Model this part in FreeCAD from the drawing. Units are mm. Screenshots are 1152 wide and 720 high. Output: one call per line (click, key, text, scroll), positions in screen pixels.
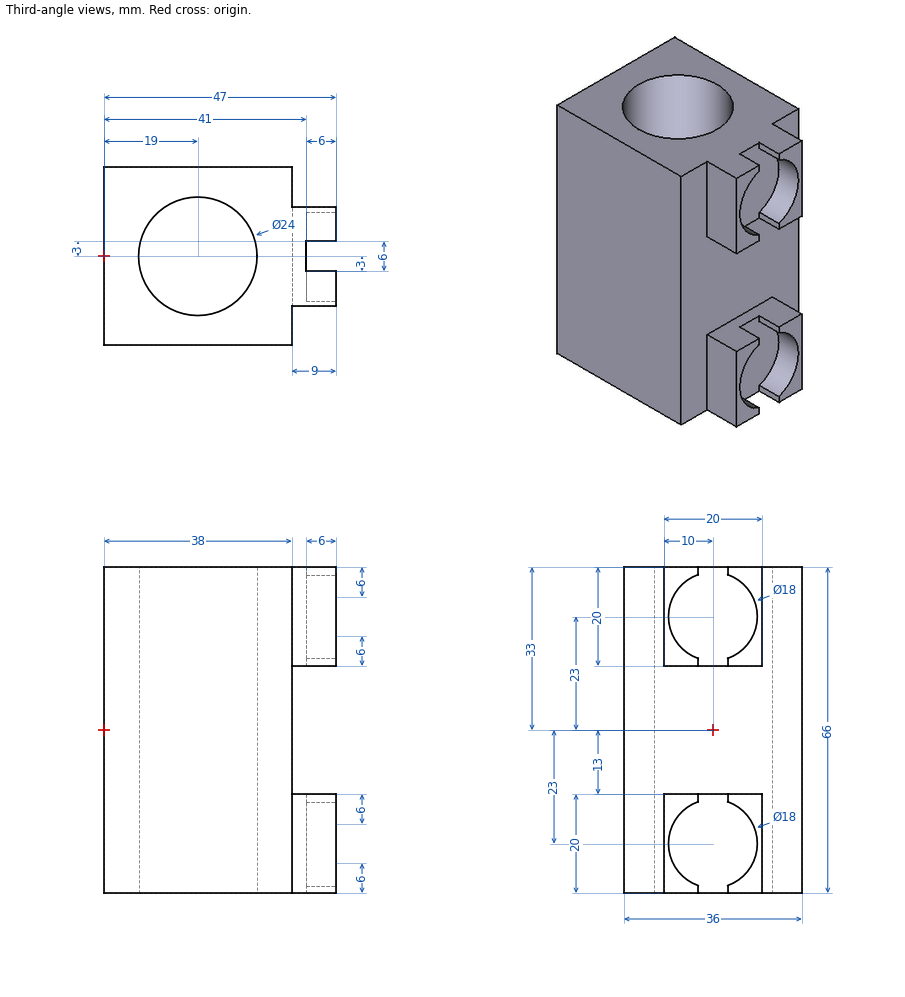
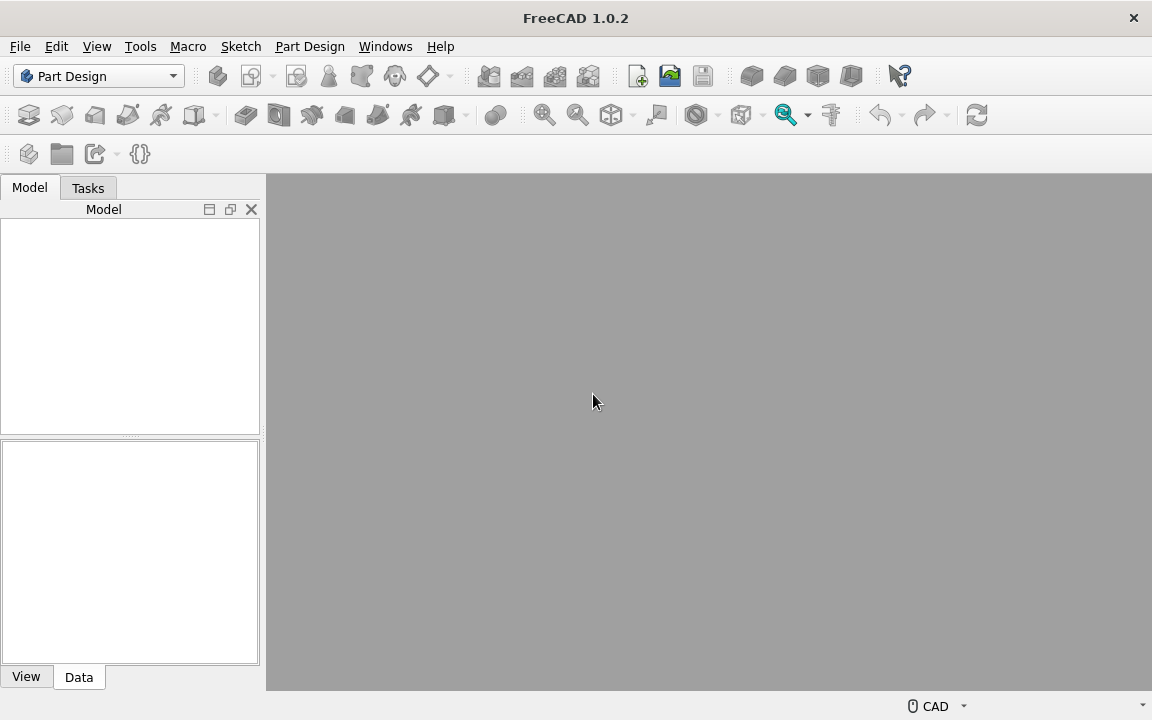
key(ctrl+n)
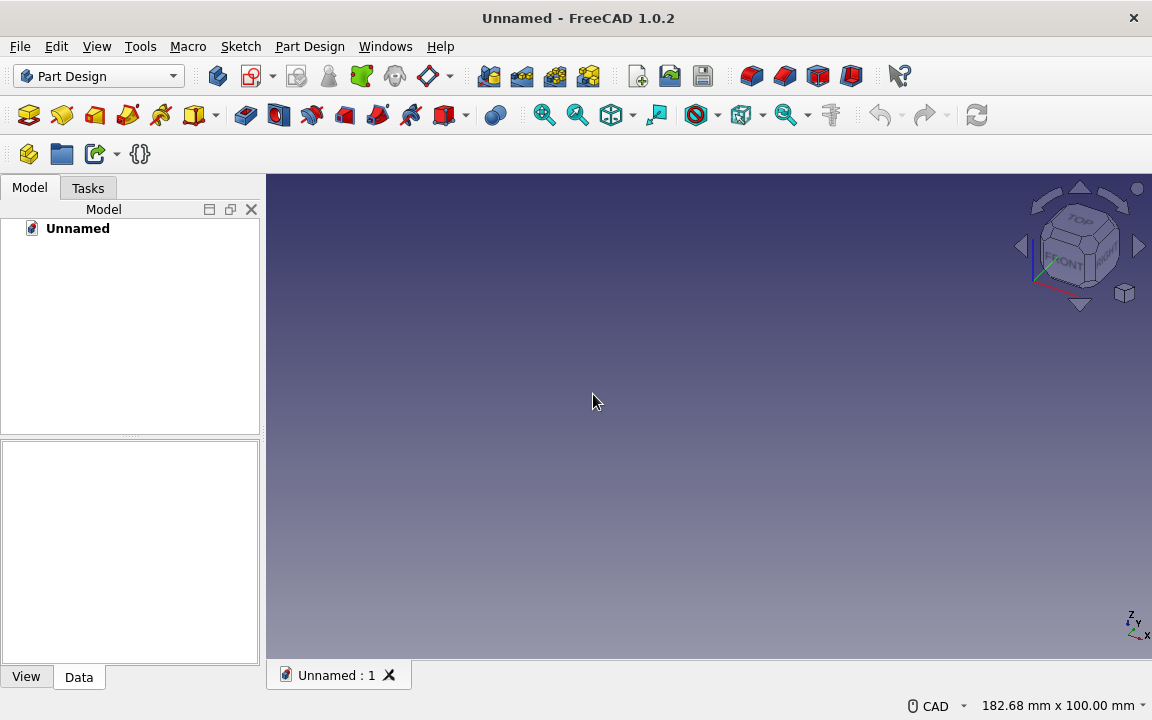
click(250, 76)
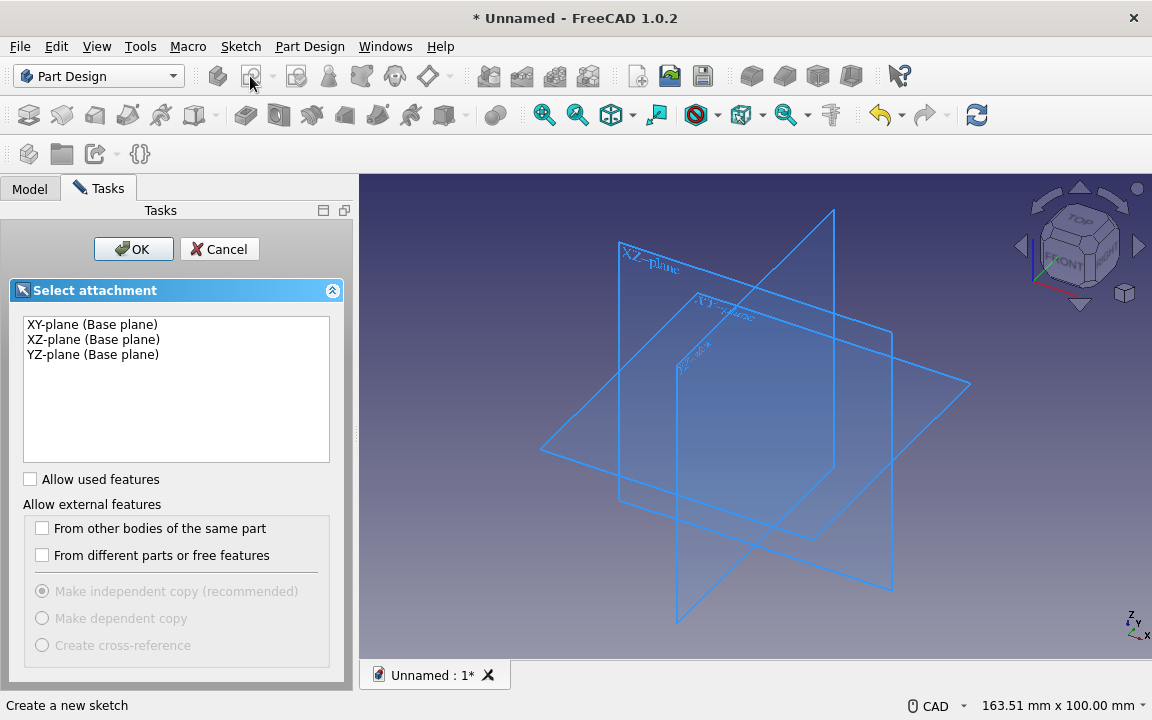
click(84, 354)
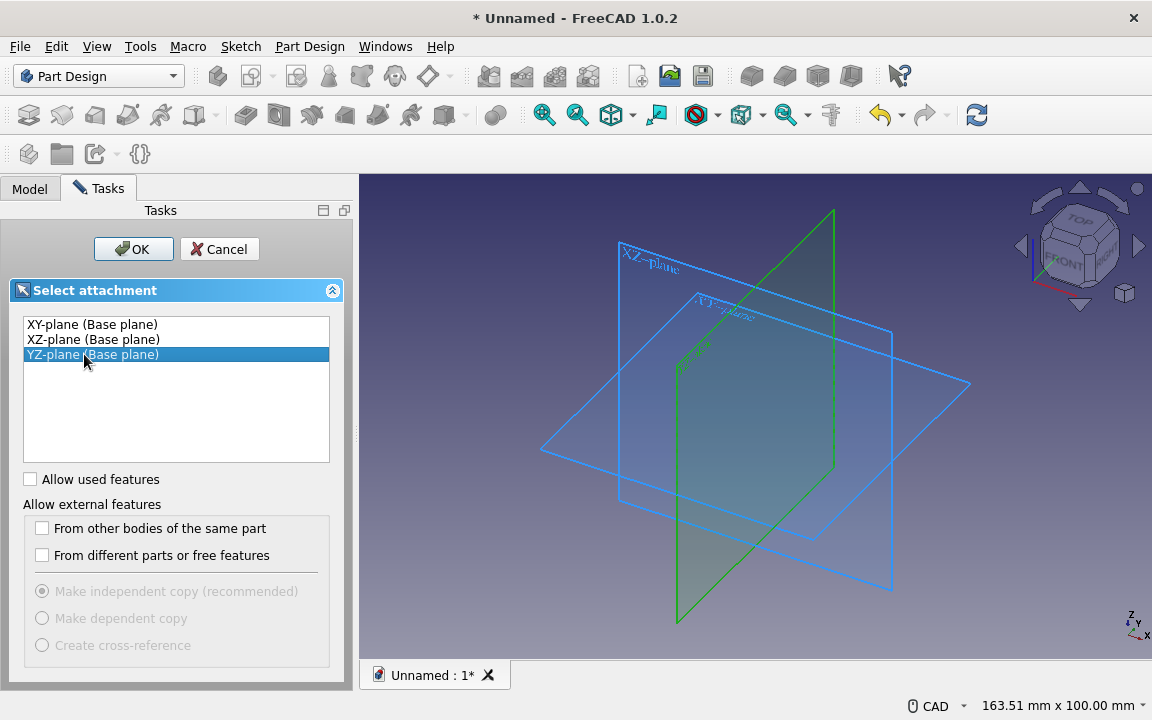
click(134, 249)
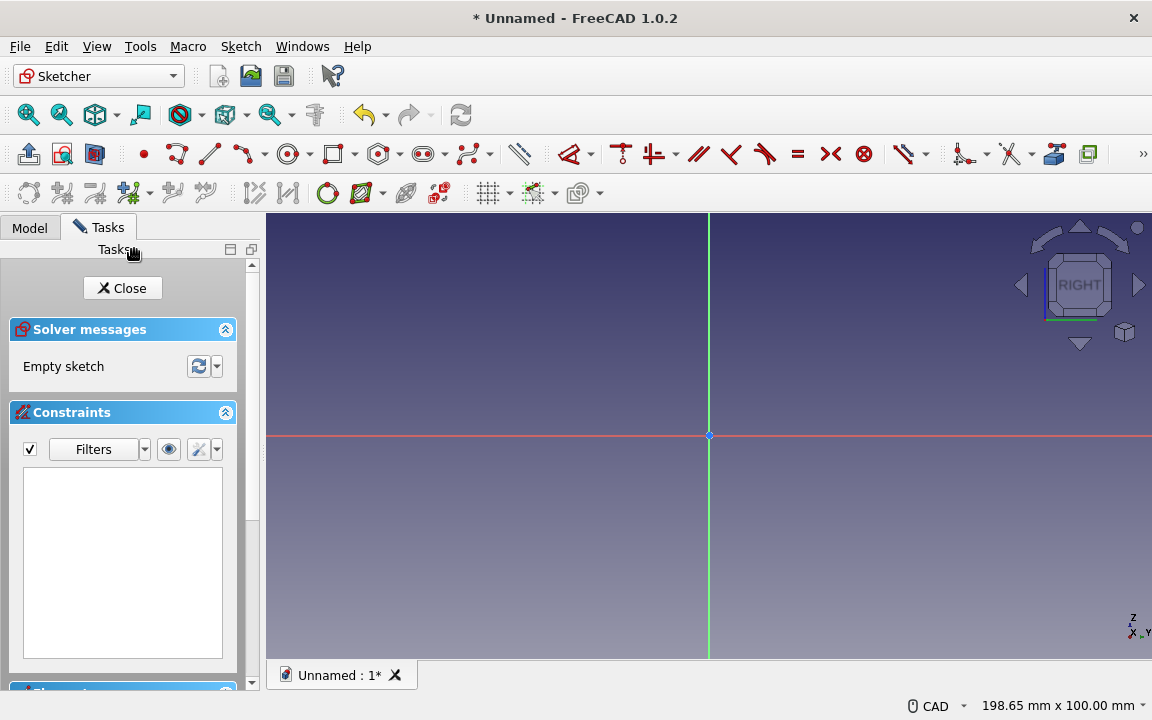
key(g)
key(v)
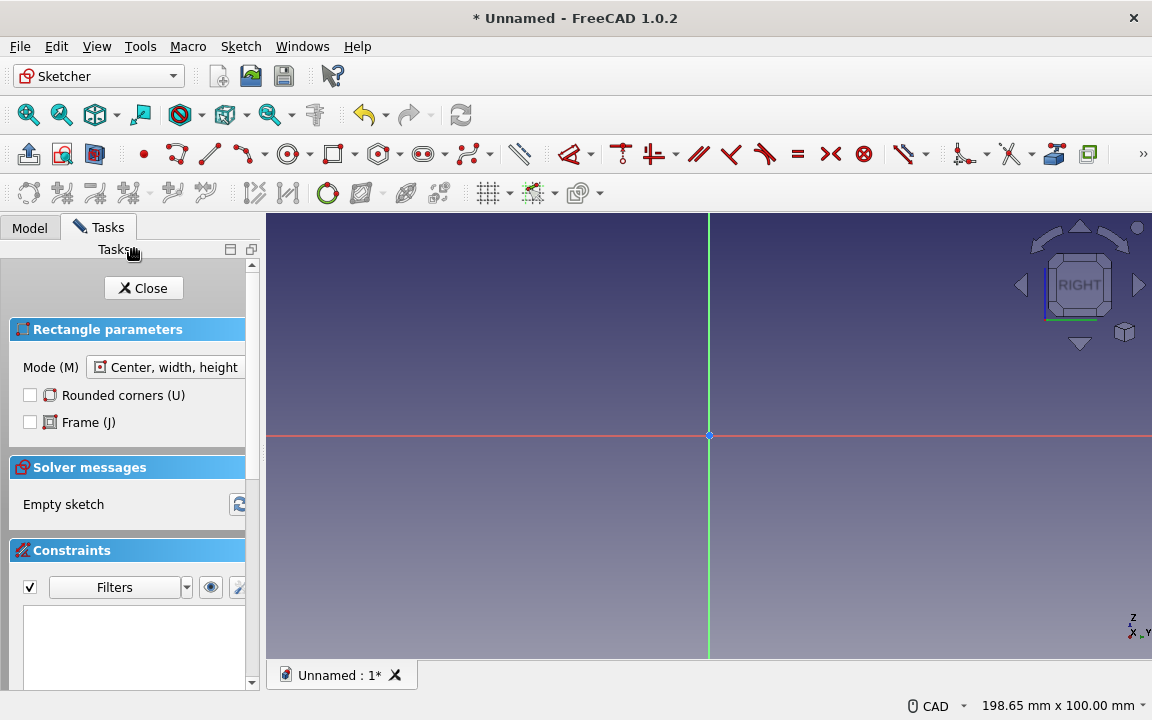
click(709, 436)
click(789, 289)
key(Escape)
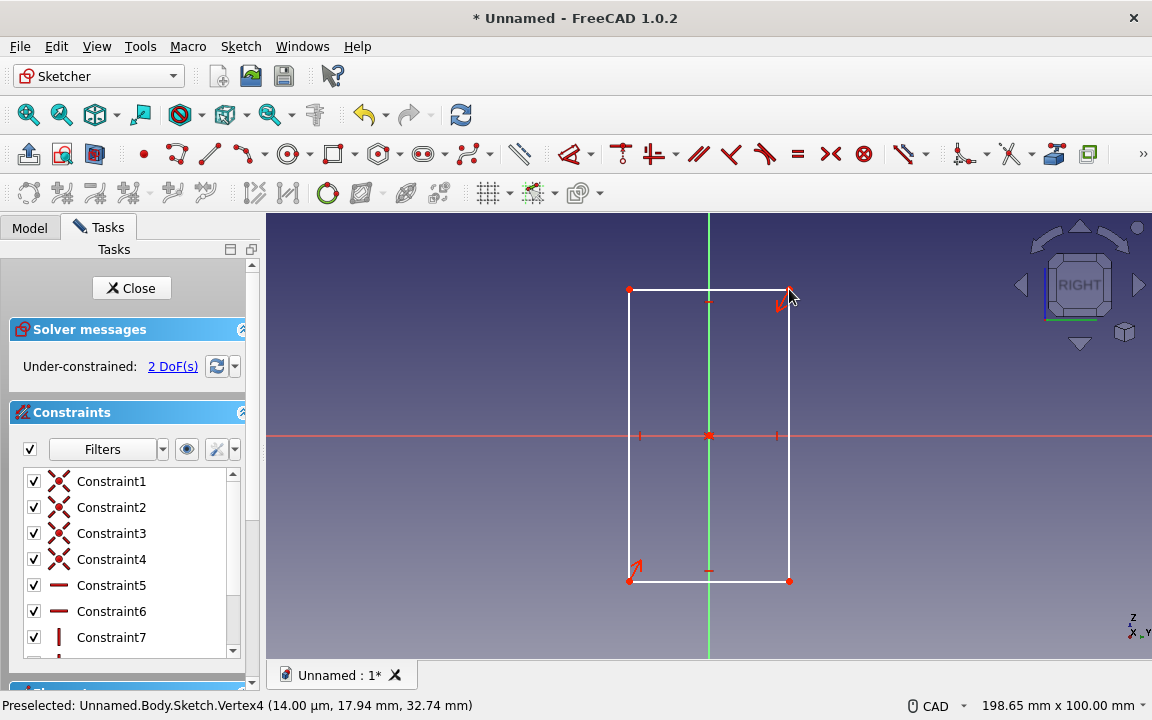
click(568, 154)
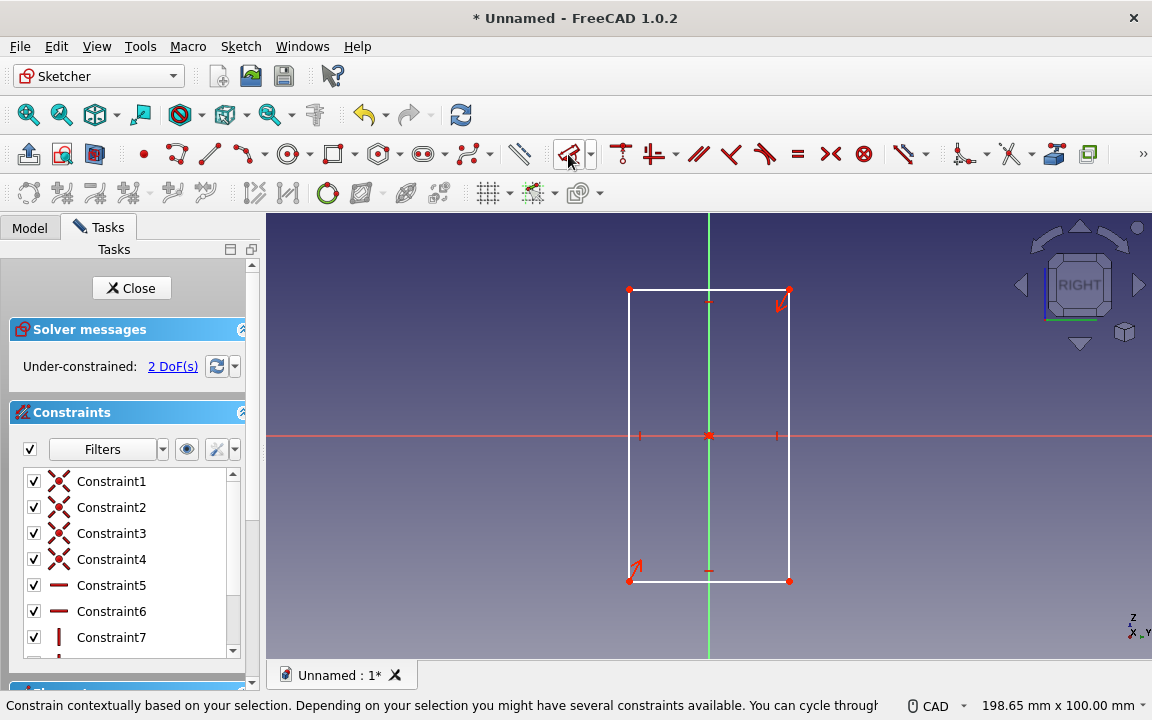
click(677, 582)
click(672, 616)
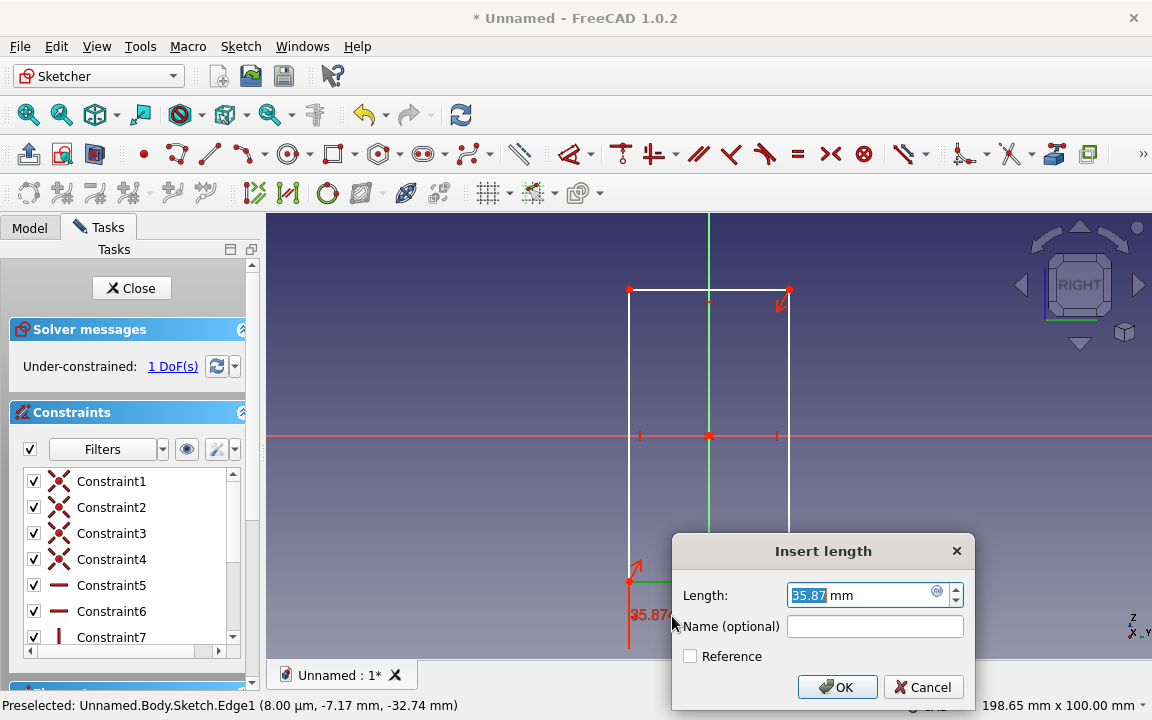
text(36)
key(Return)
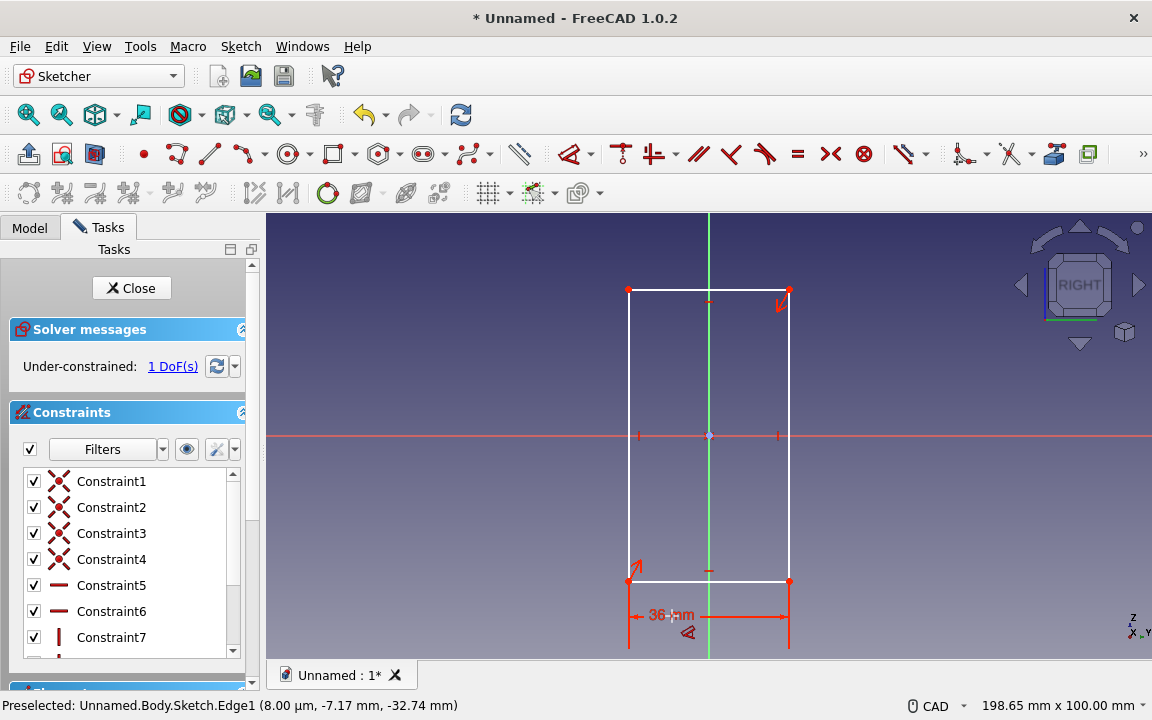
click(789, 494)
click(823, 369)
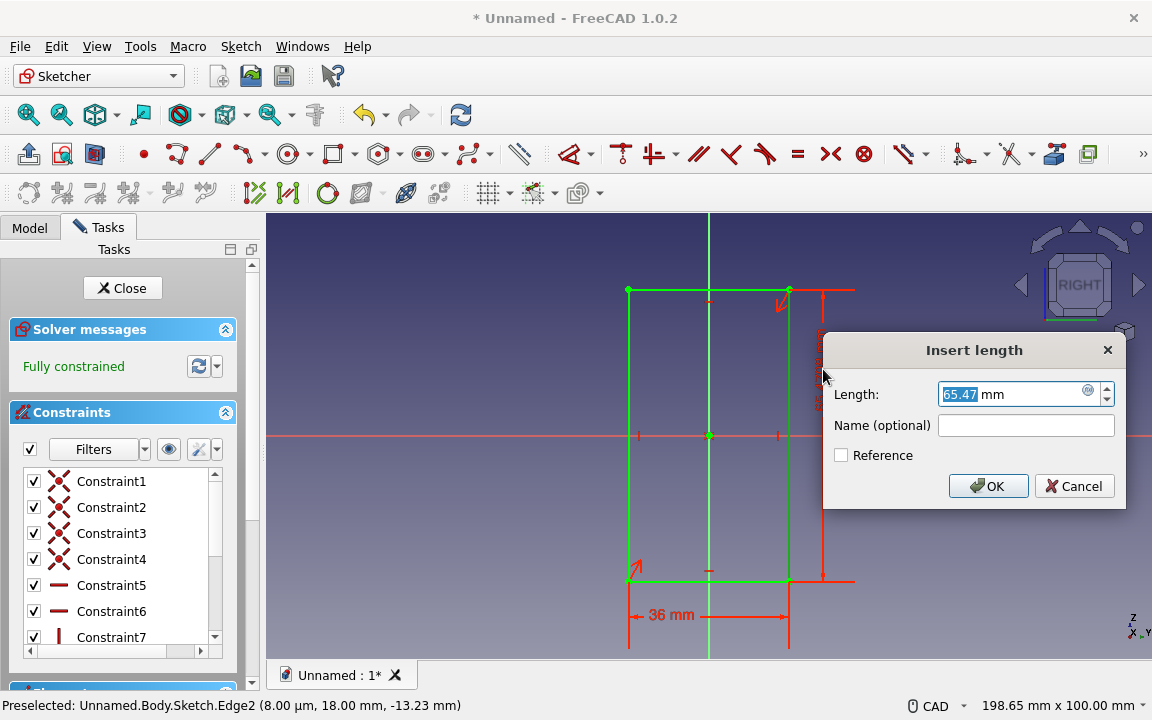
text(66)
key(Return)
key(Escape)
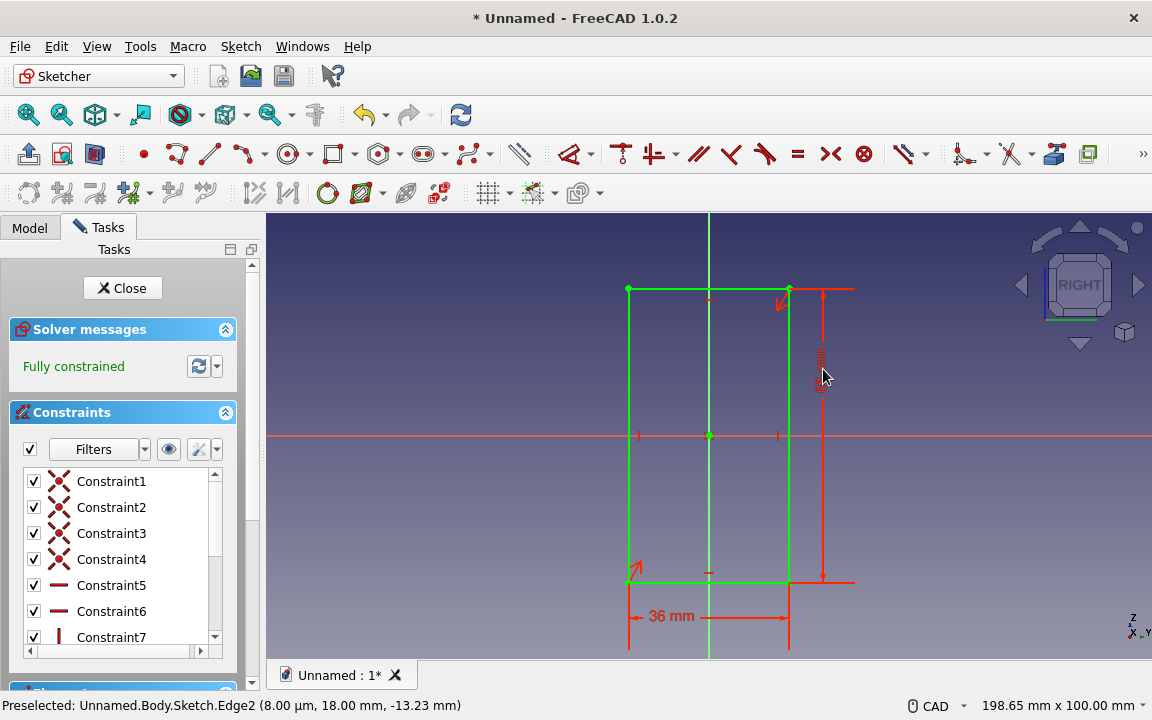
click(123, 288)